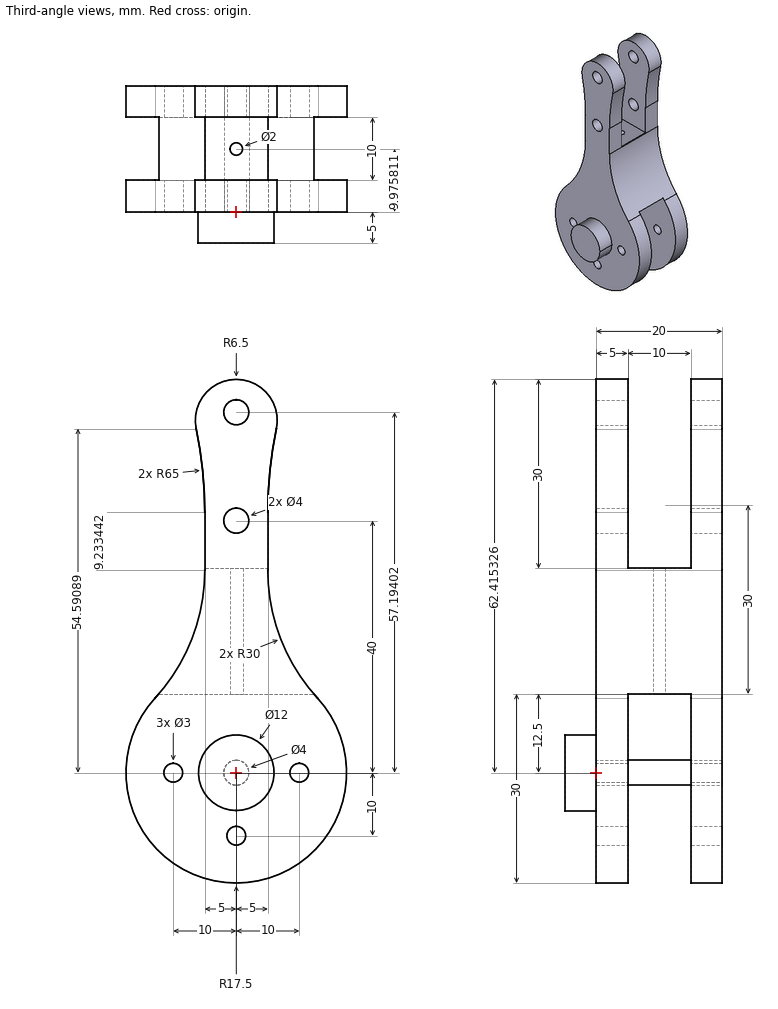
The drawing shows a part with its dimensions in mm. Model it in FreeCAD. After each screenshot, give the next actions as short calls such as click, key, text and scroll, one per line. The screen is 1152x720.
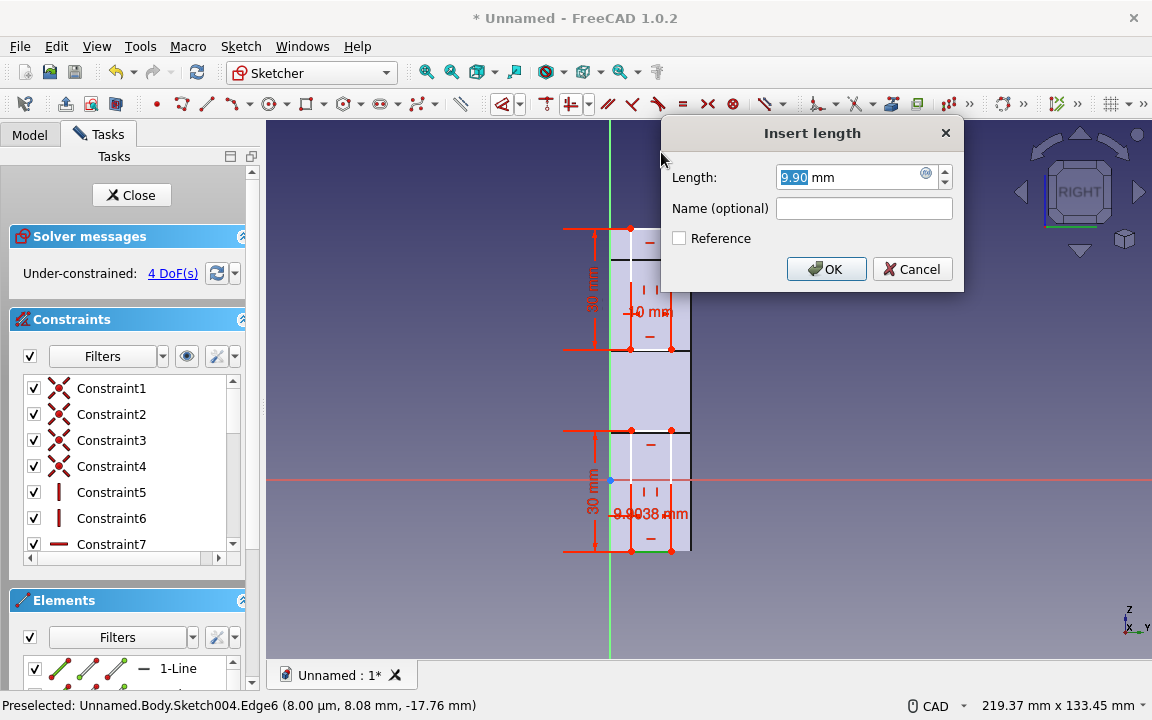
text(10)
key(Return)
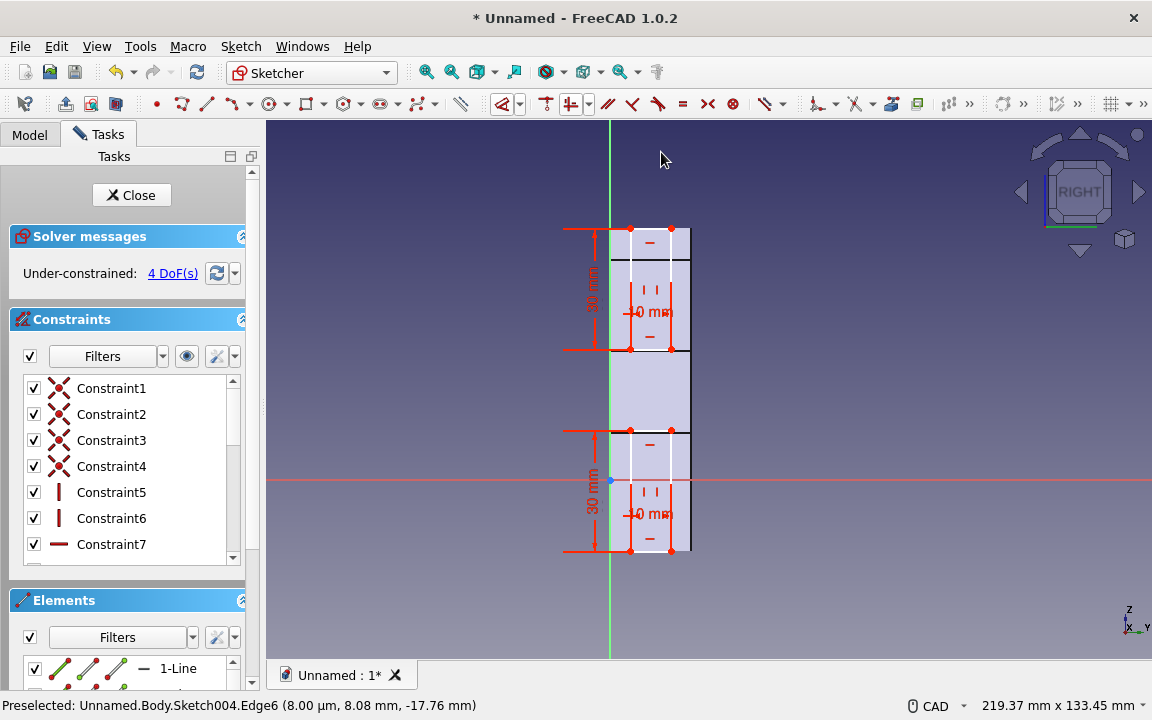
scroll(631, 229, up, 4)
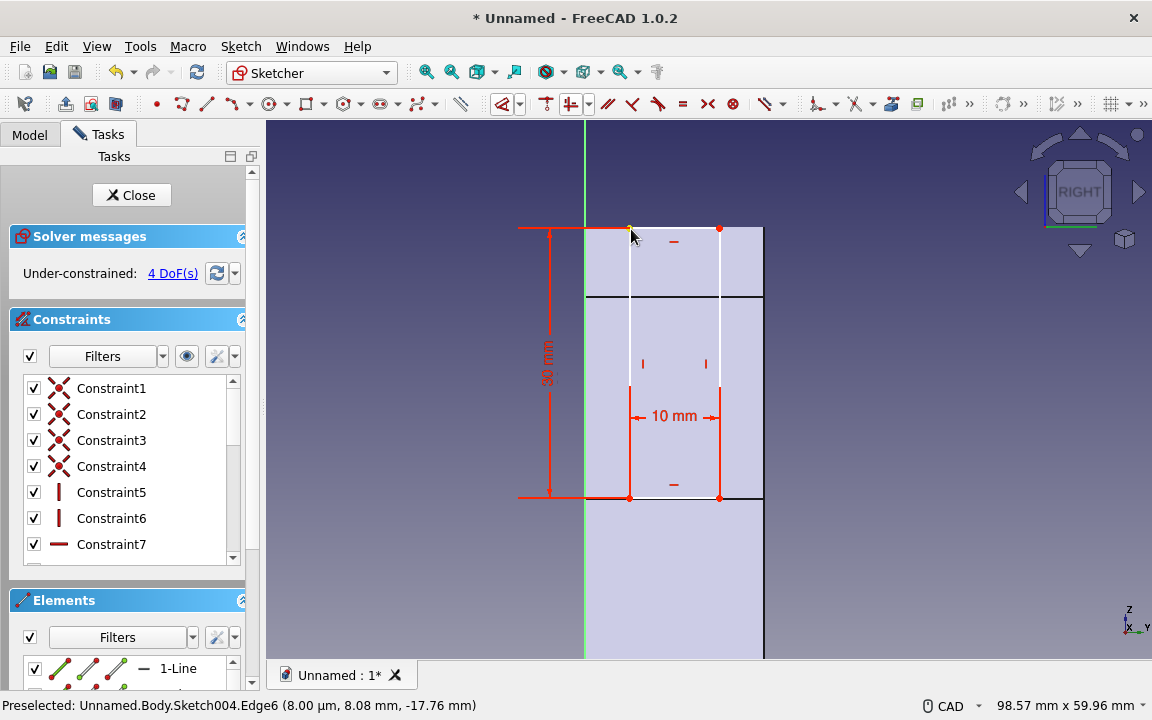
click(630, 228)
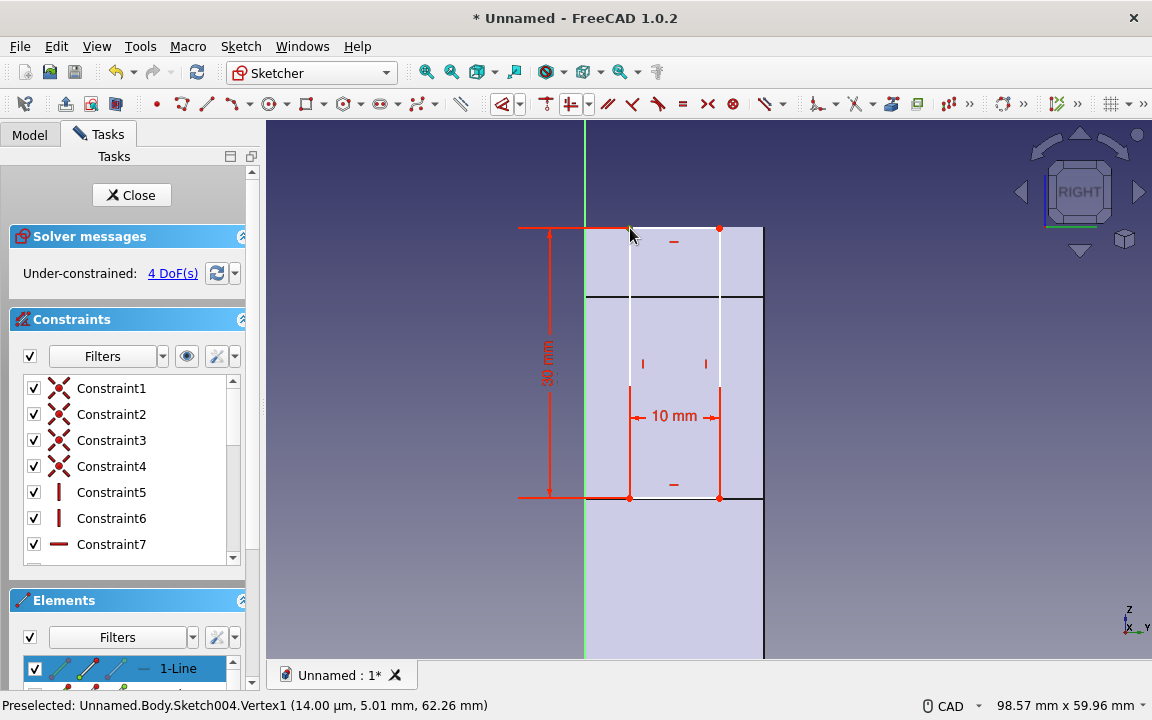
key(l)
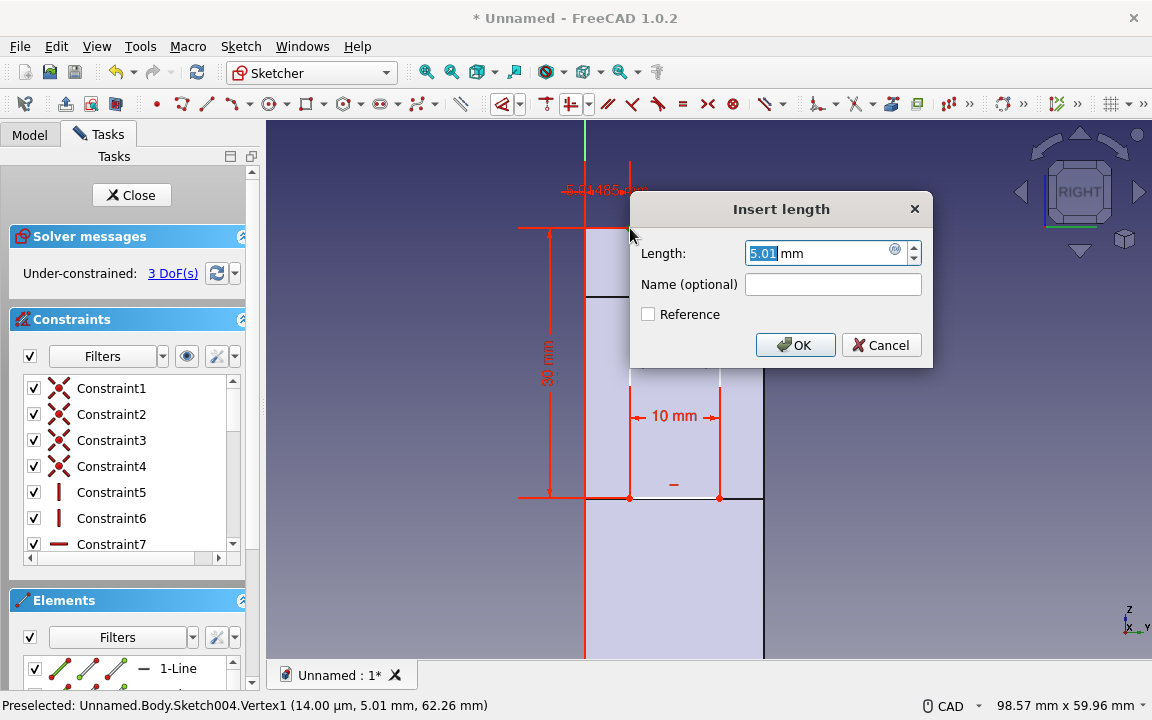
text(5)
key(Return)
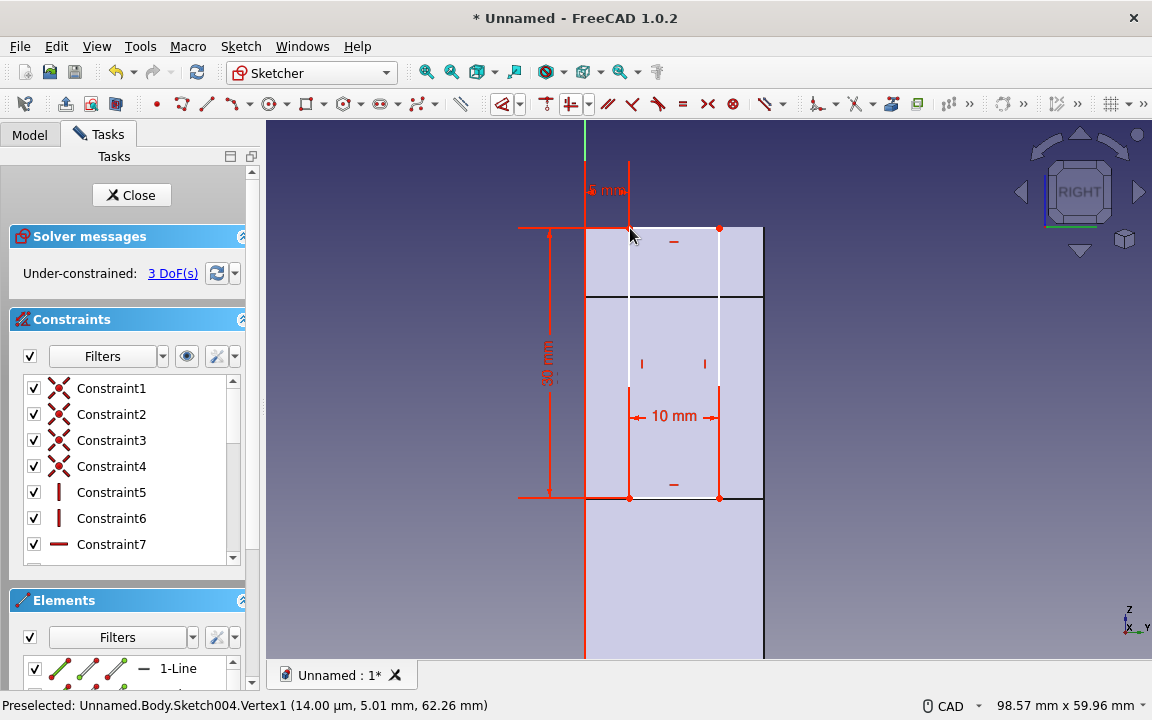
scroll(631, 229, down, 4)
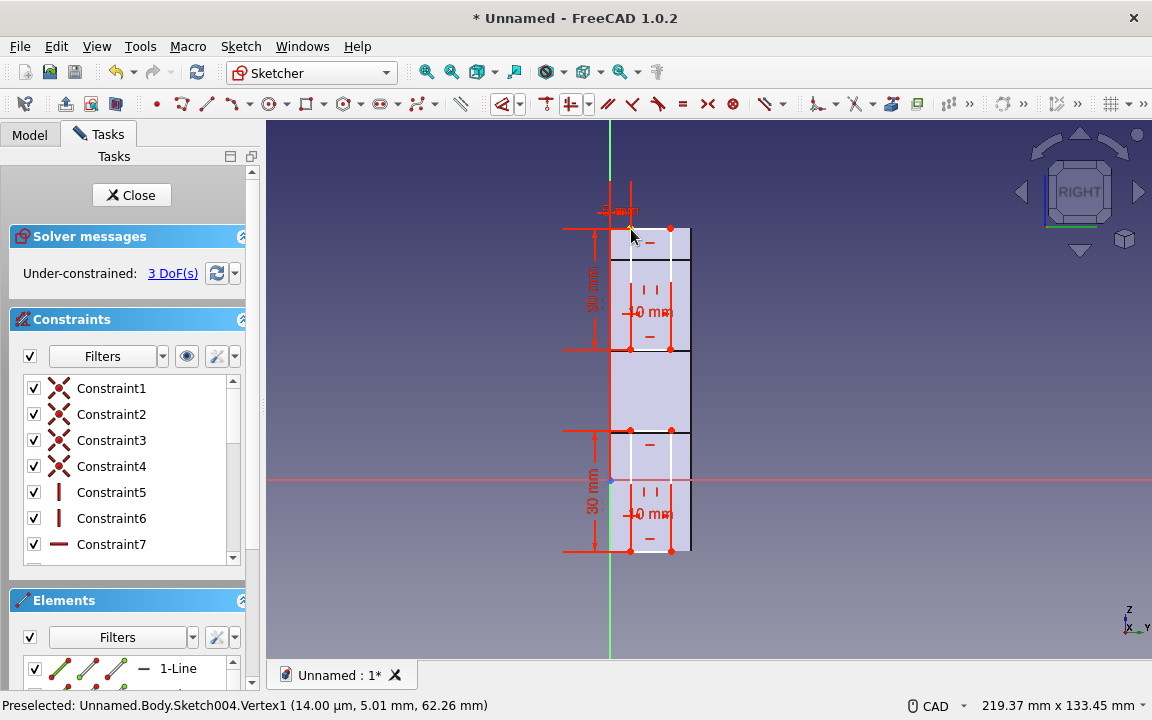
scroll(631, 431, up, 4)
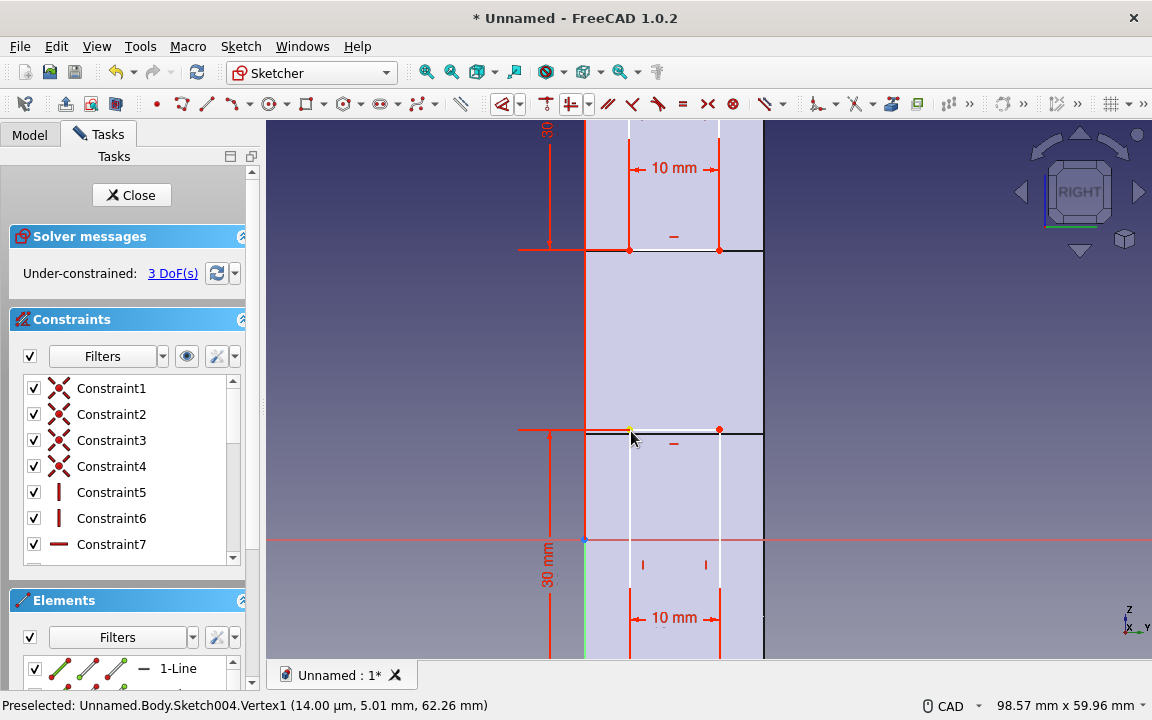
click(630, 430)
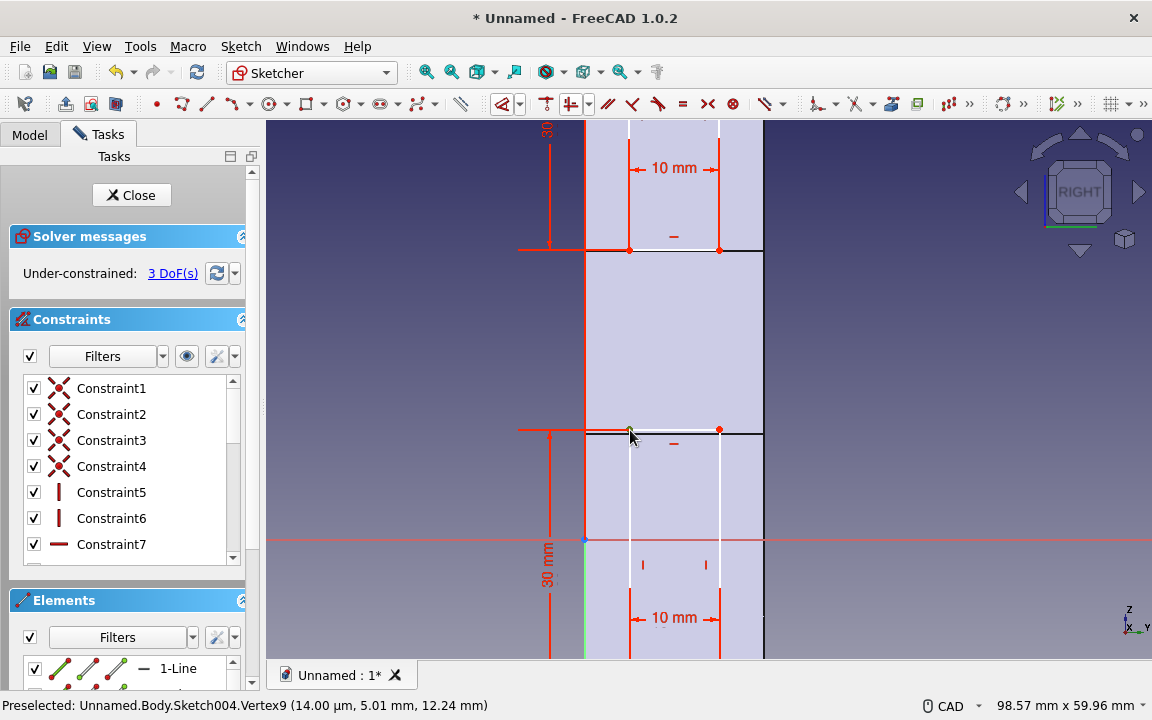
key(l)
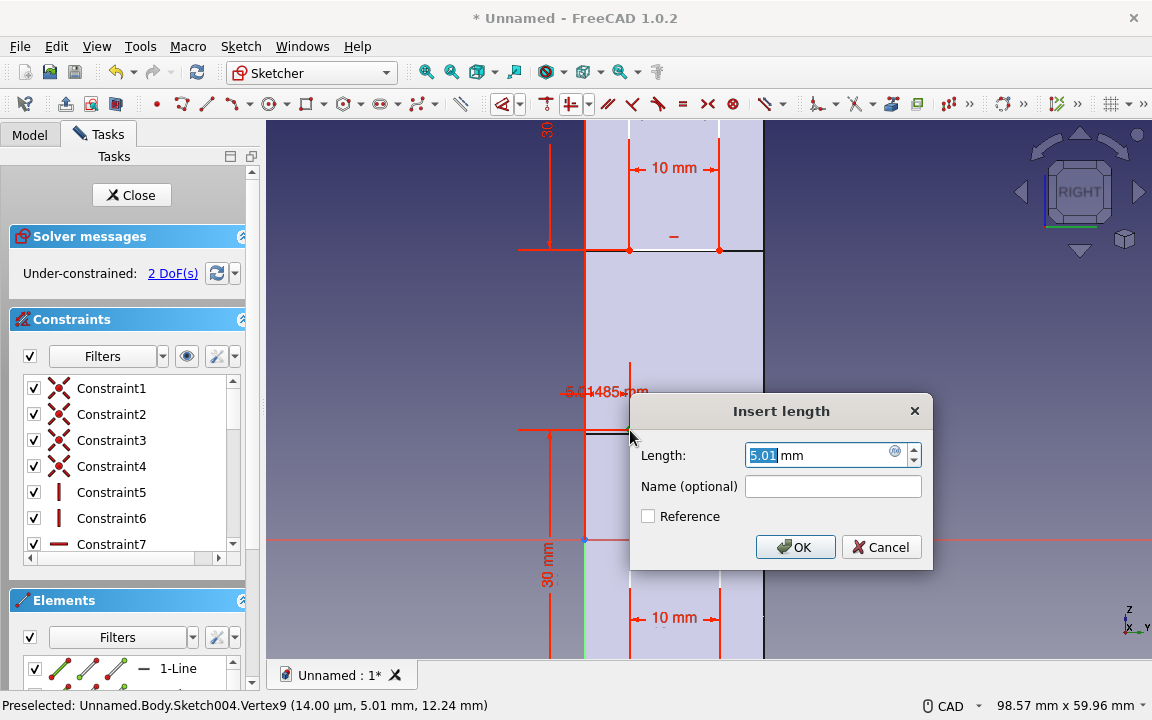
text(5)
key(Return)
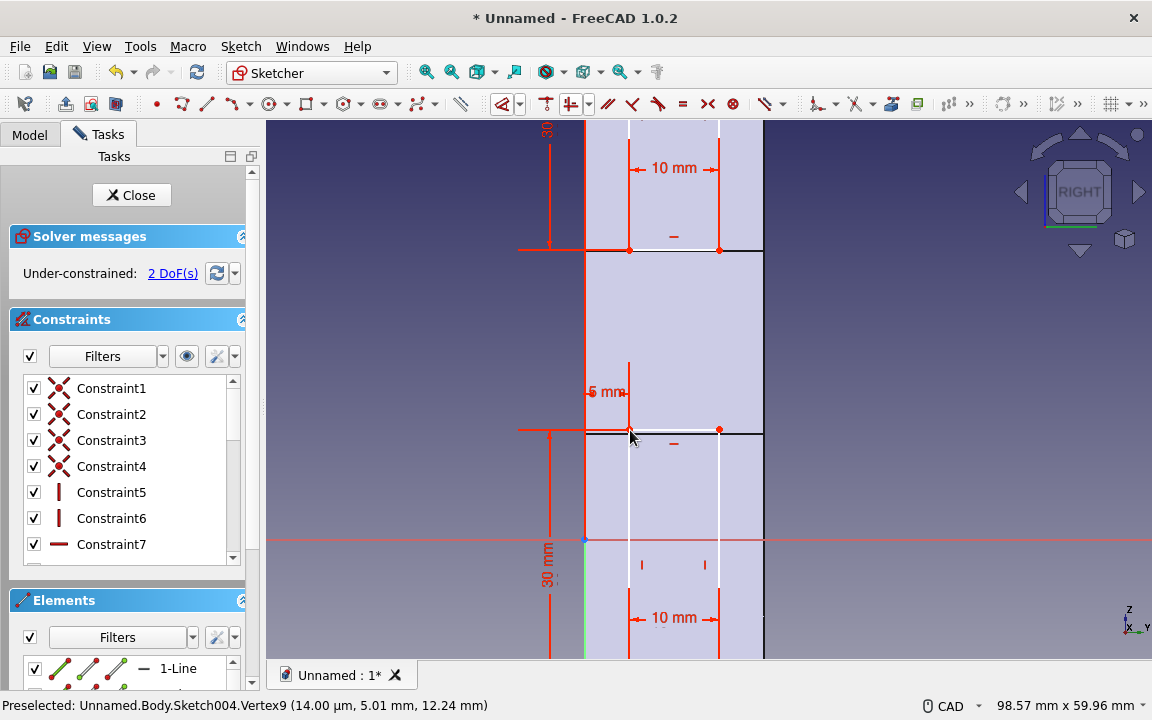
click(629, 430)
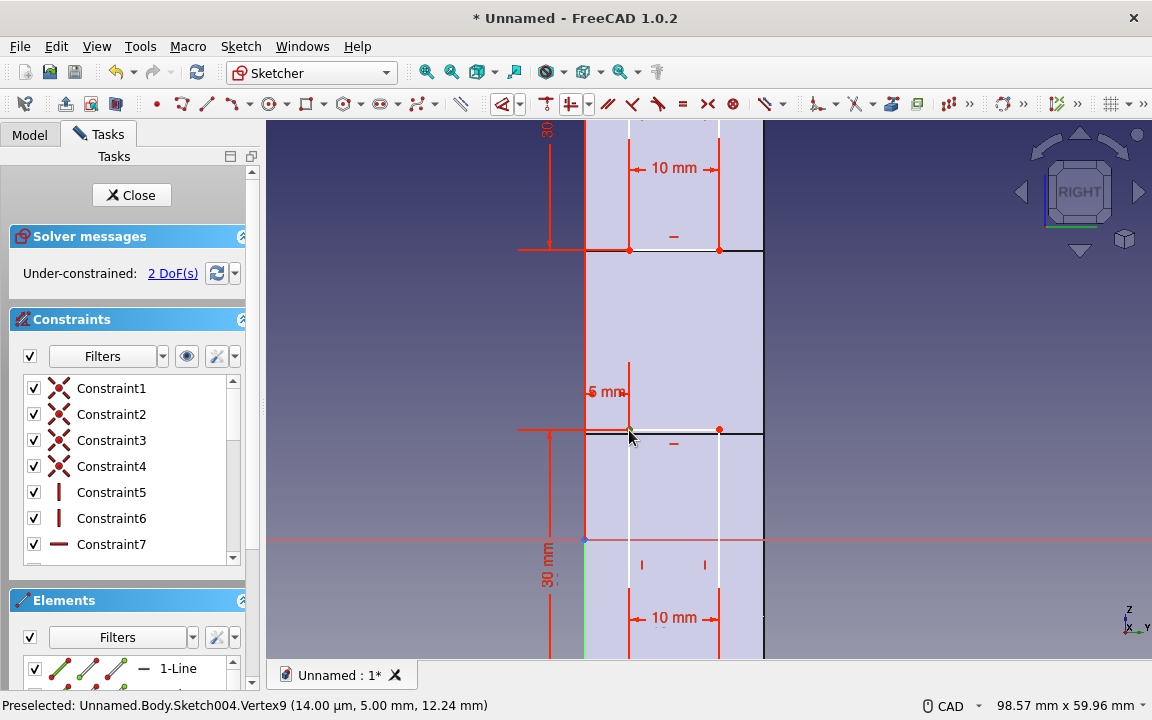
key(i)